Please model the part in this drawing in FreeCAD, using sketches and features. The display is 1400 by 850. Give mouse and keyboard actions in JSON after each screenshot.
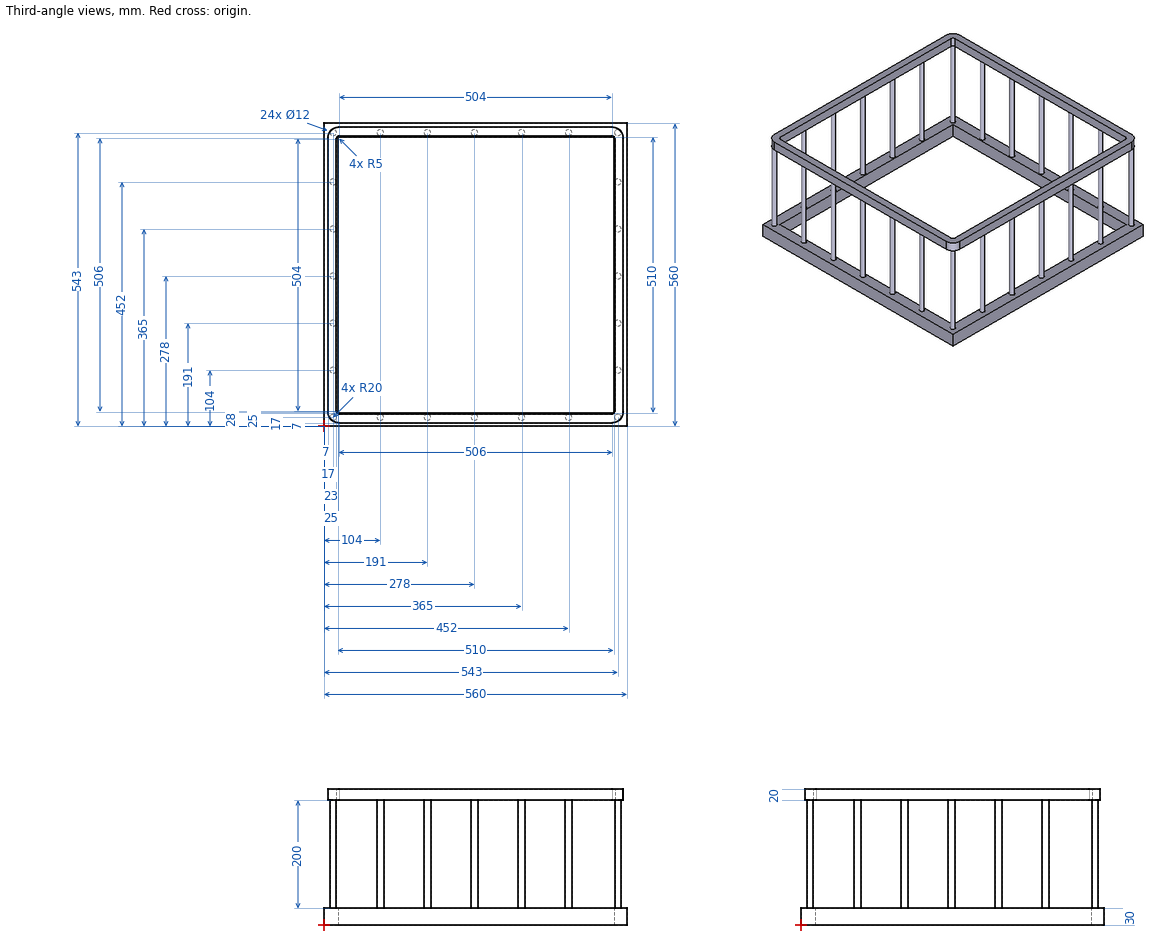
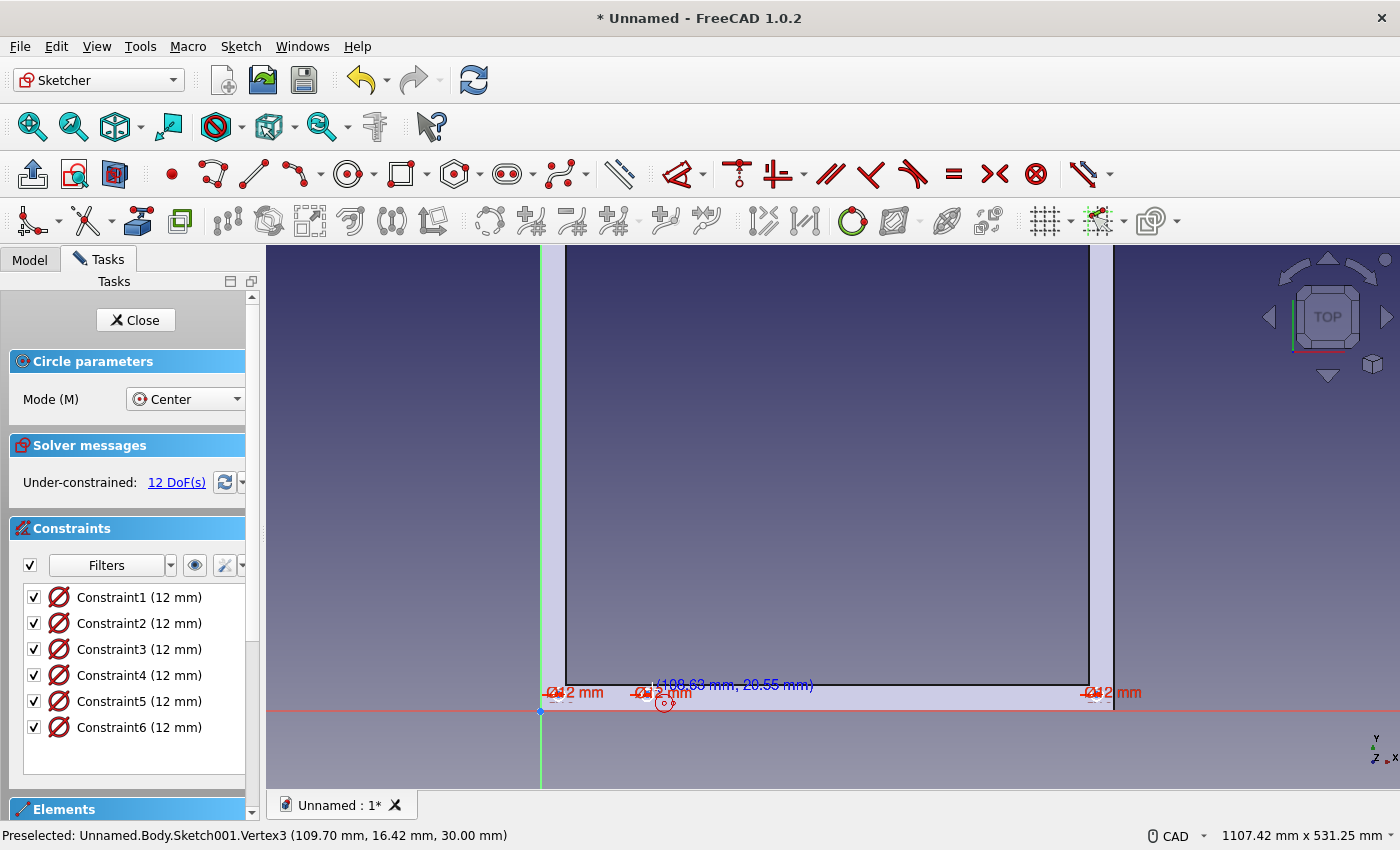
{"action": "scroll", "coordinate": [648, 694], "scroll_direction": "down", "scroll_amount": 2}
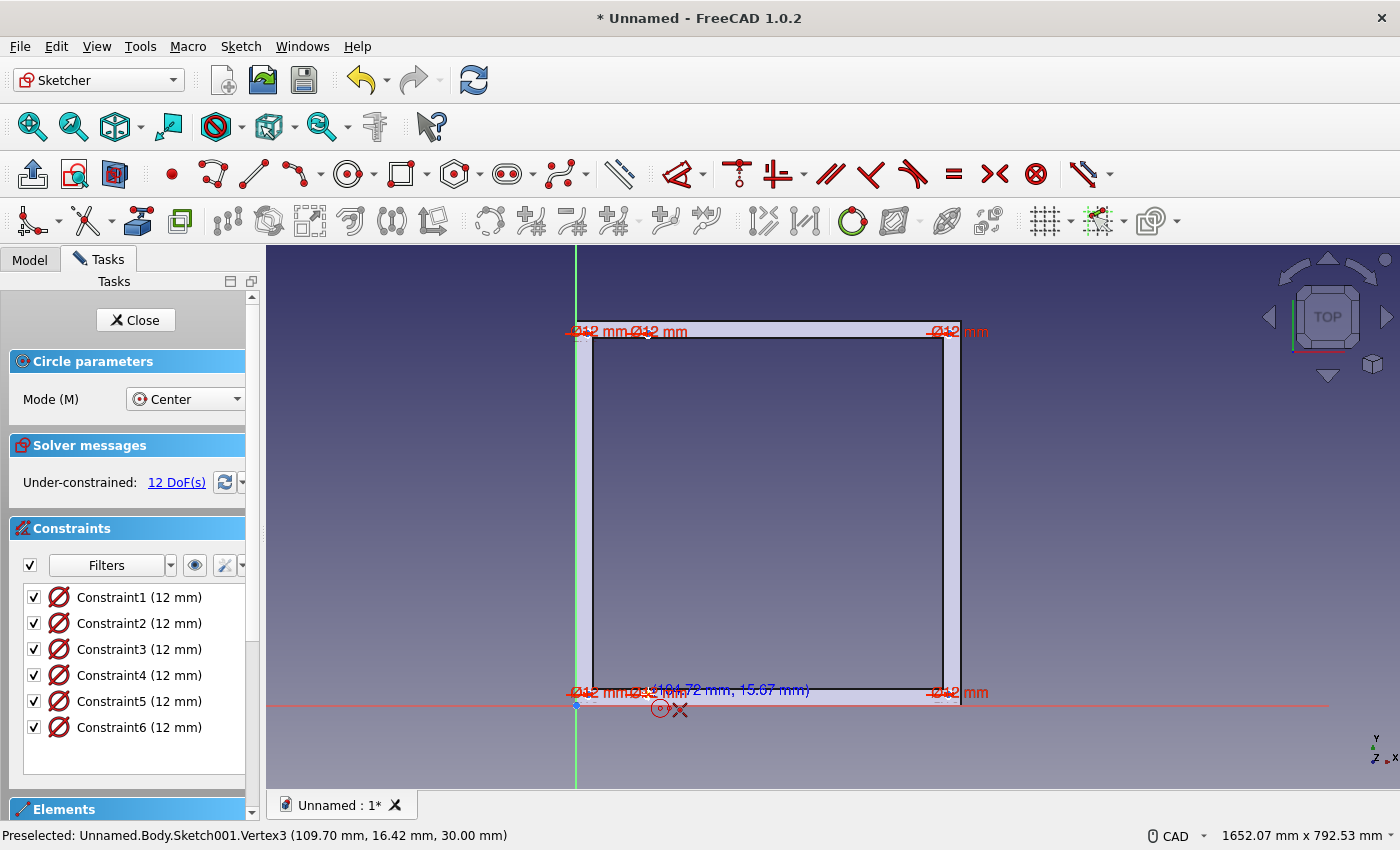
{"action": "scroll", "coordinate": [707, 333], "scroll_direction": "up", "scroll_amount": 9}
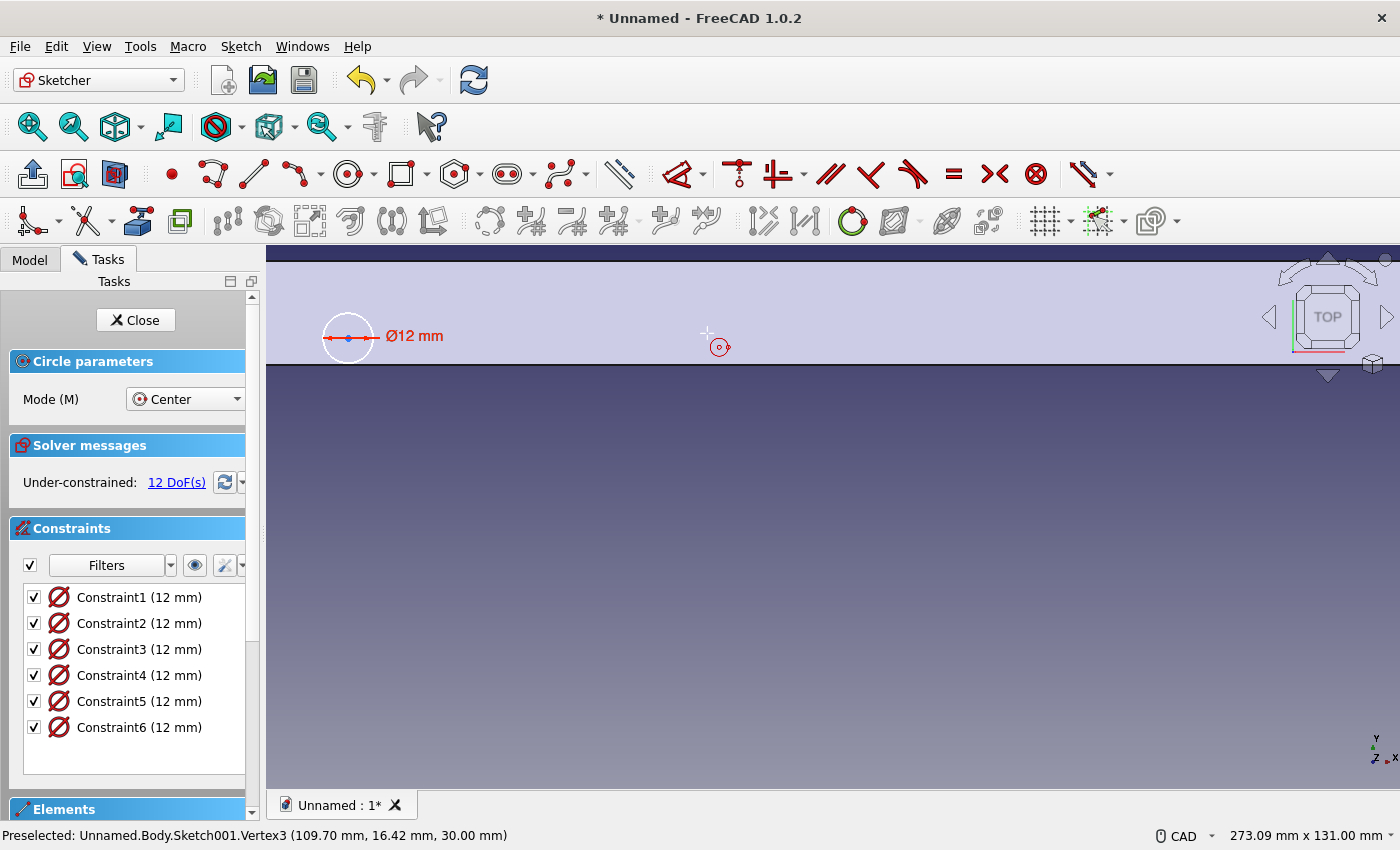
{"action": "scroll", "coordinate": [707, 333], "scroll_direction": "down", "scroll_amount": 9}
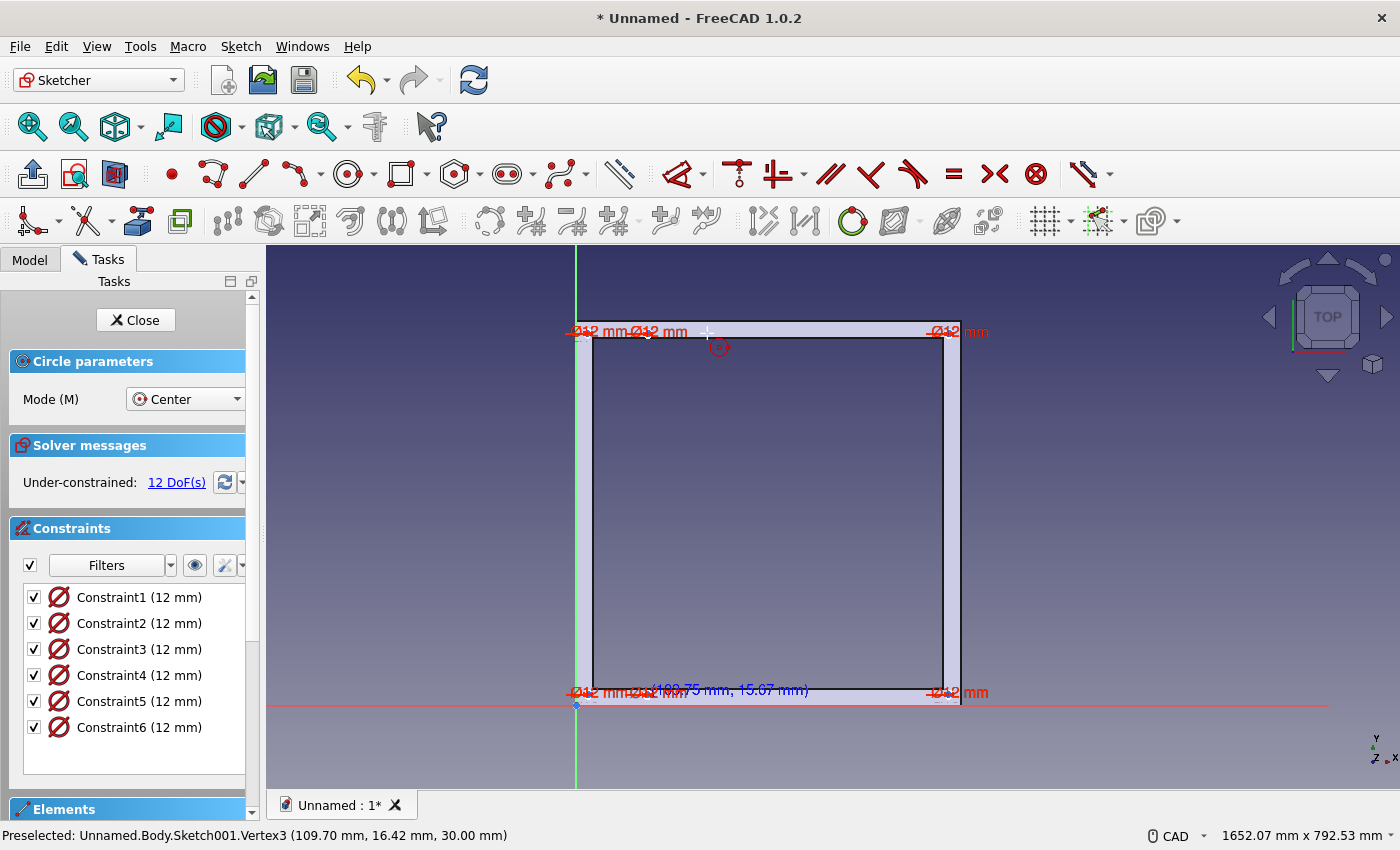
{"action": "left_click", "coordinate": [707, 333]}
{"action": "mouse_move", "coordinate": [710, 330]}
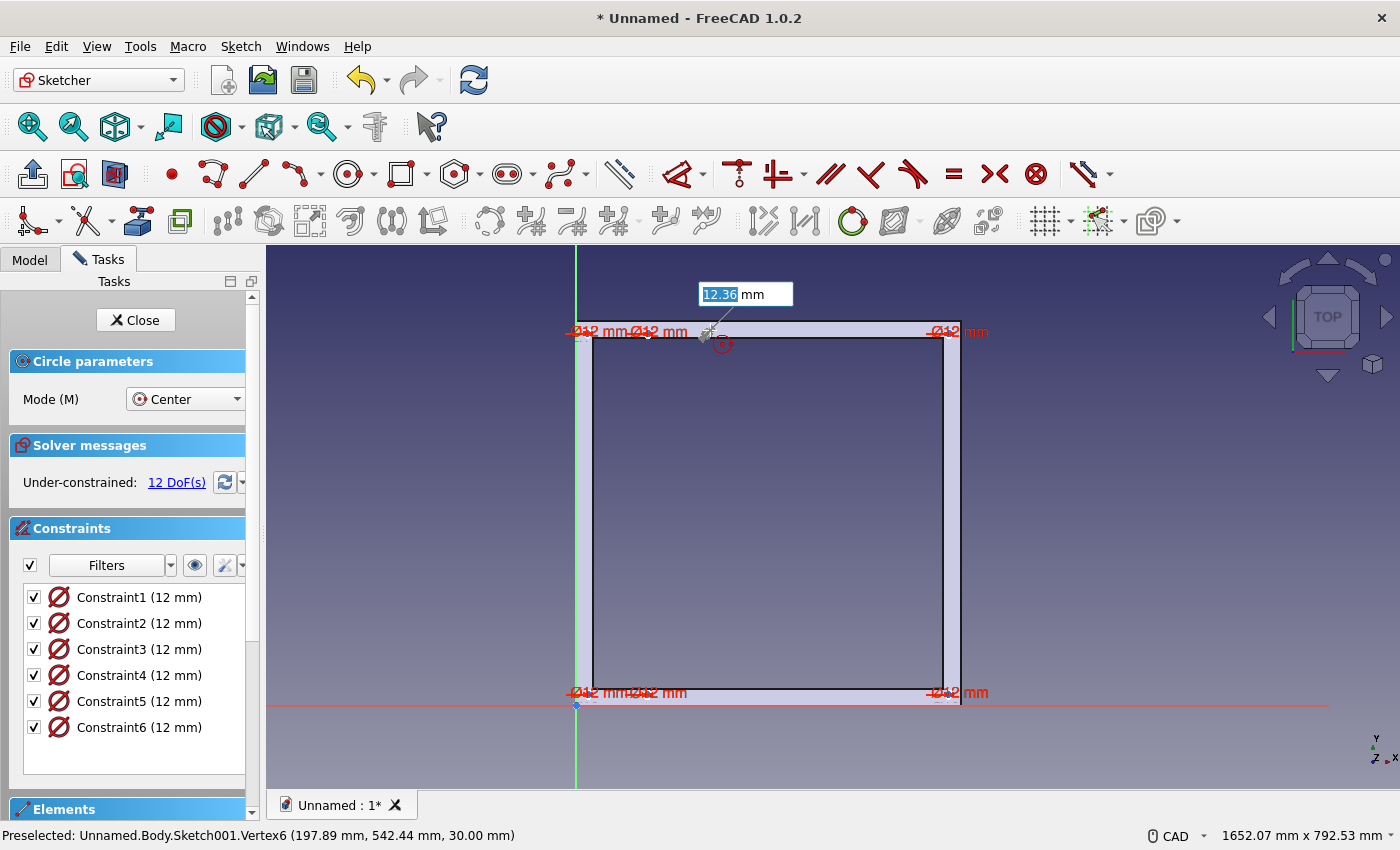
{"action": "type", "text": "12"}
{"action": "key", "text": "Return"}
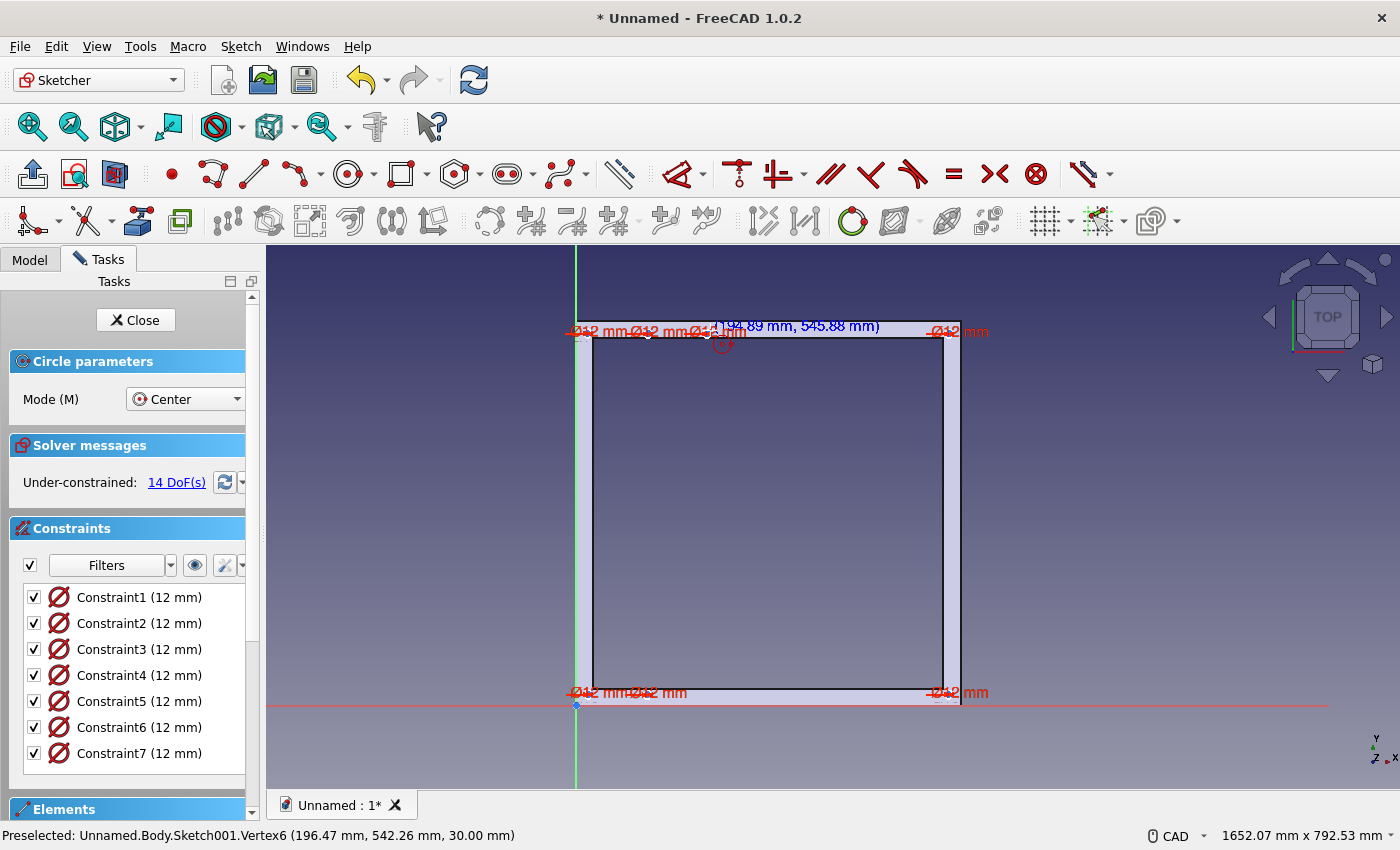
{"action": "scroll", "coordinate": [707, 694], "scroll_direction": "up", "scroll_amount": 9}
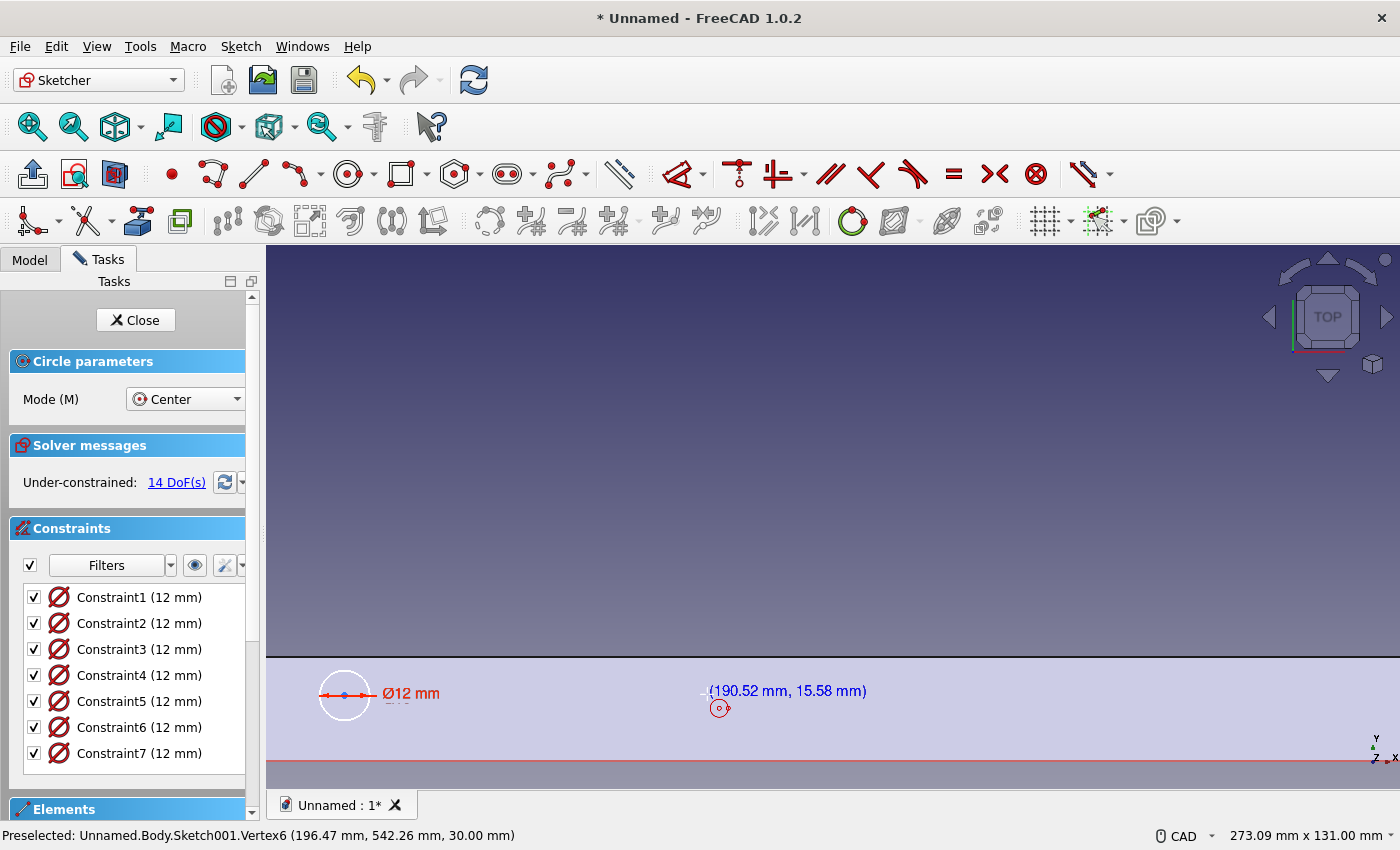
{"action": "scroll", "coordinate": [707, 694], "scroll_direction": "down", "scroll_amount": 9}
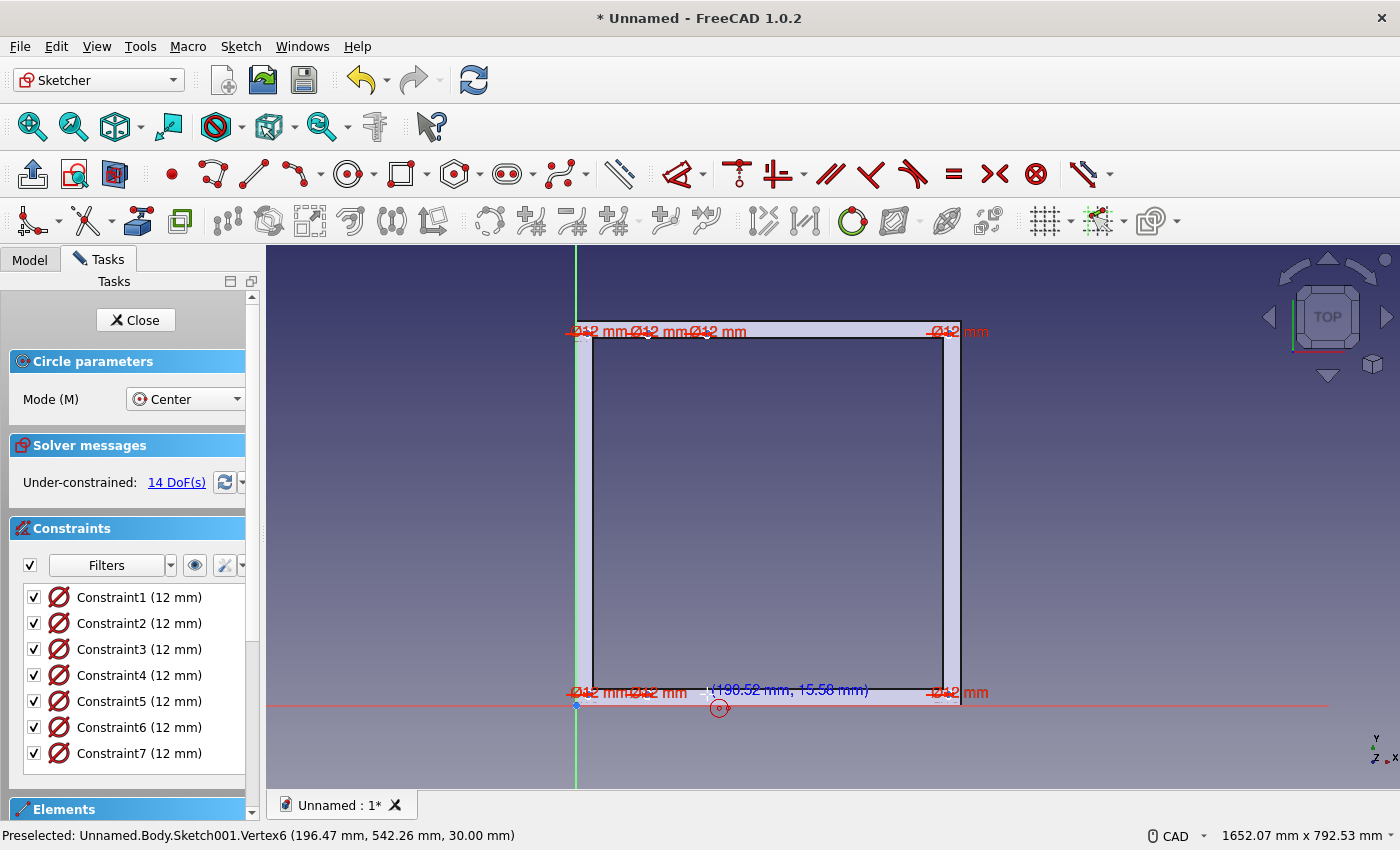
{"action": "scroll", "coordinate": [707, 694], "scroll_direction": "up", "scroll_amount": 2}